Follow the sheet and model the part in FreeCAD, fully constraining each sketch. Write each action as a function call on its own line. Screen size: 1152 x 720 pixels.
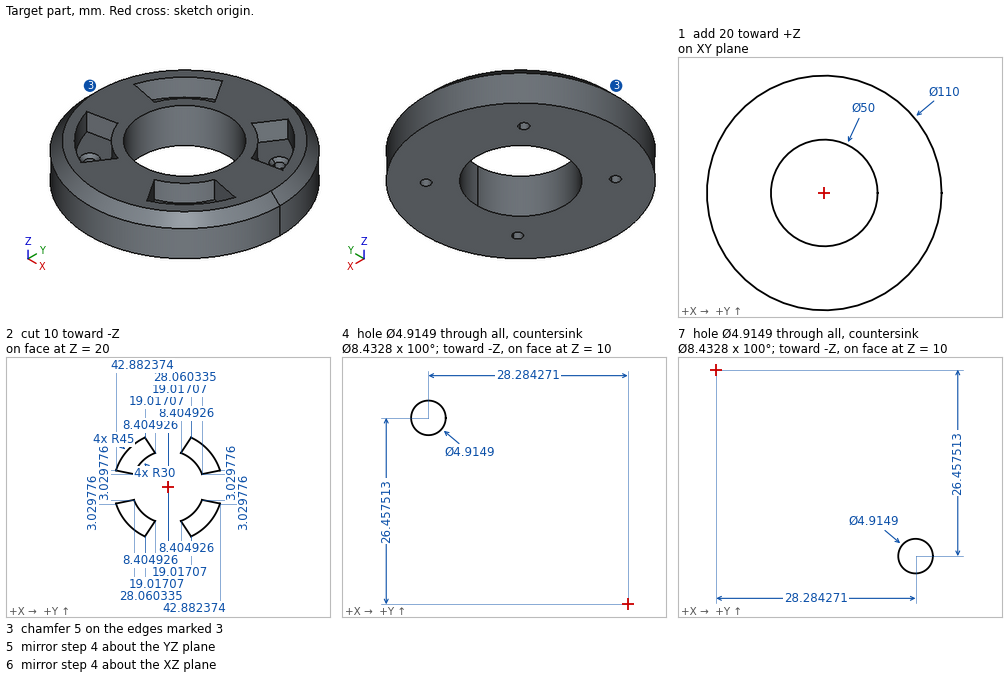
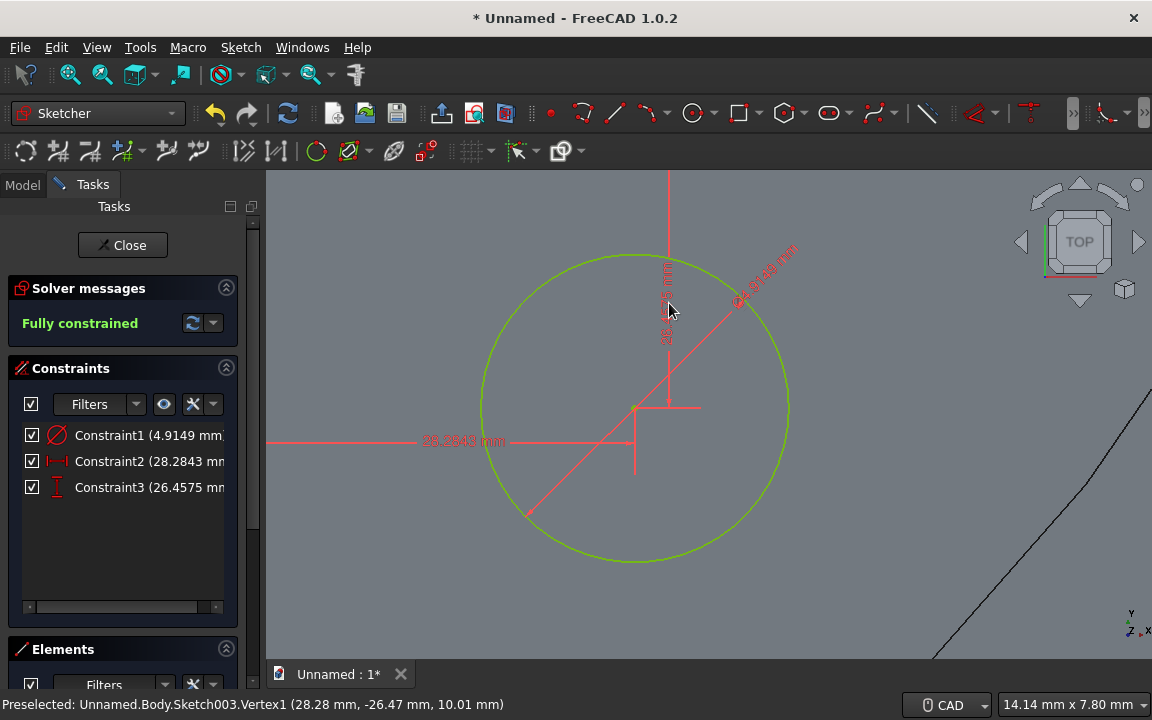
click(123, 245)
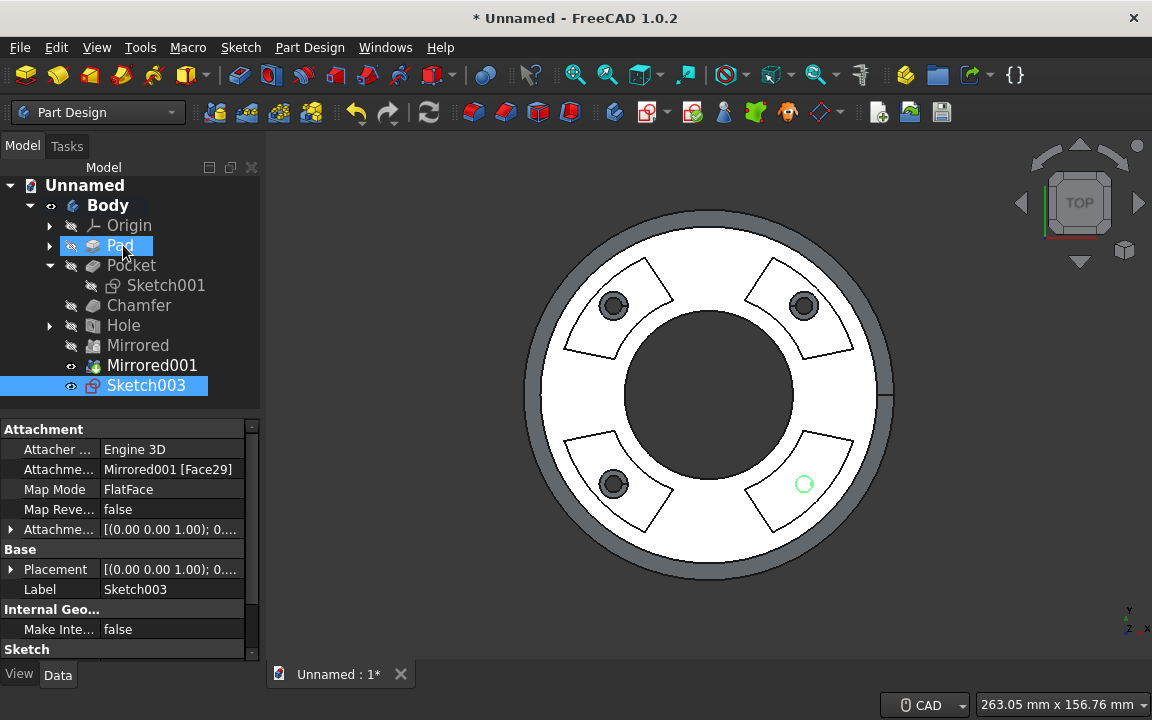
click(272, 76)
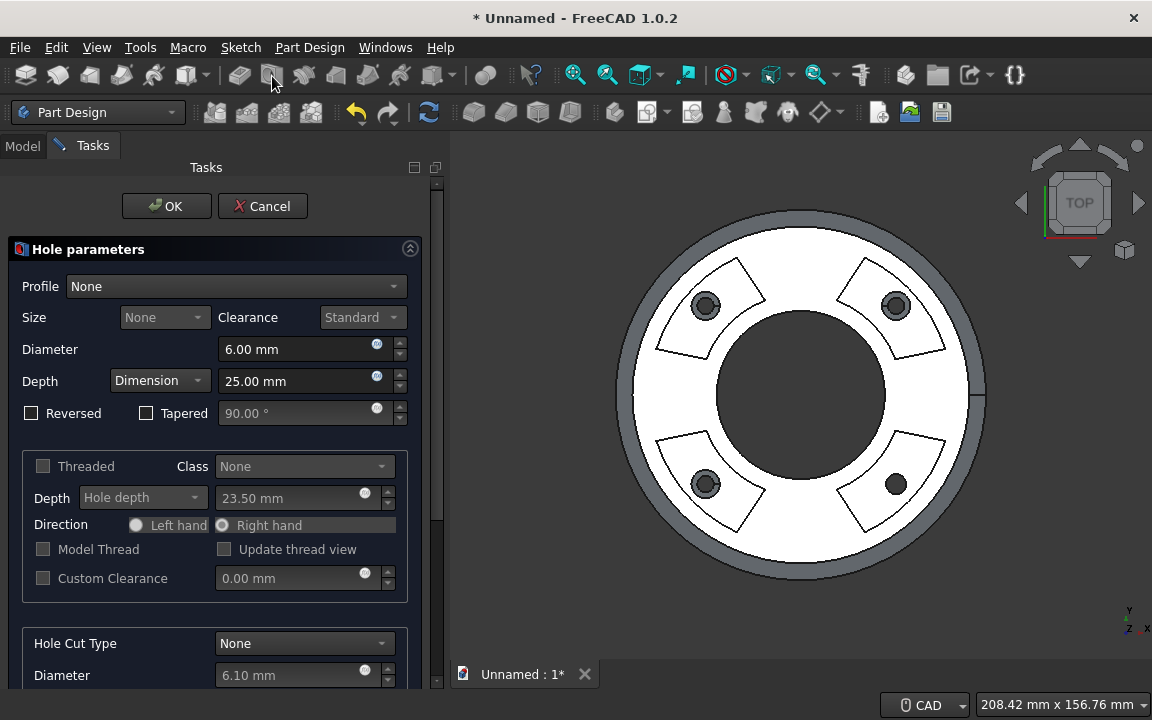
triple_click(305, 349)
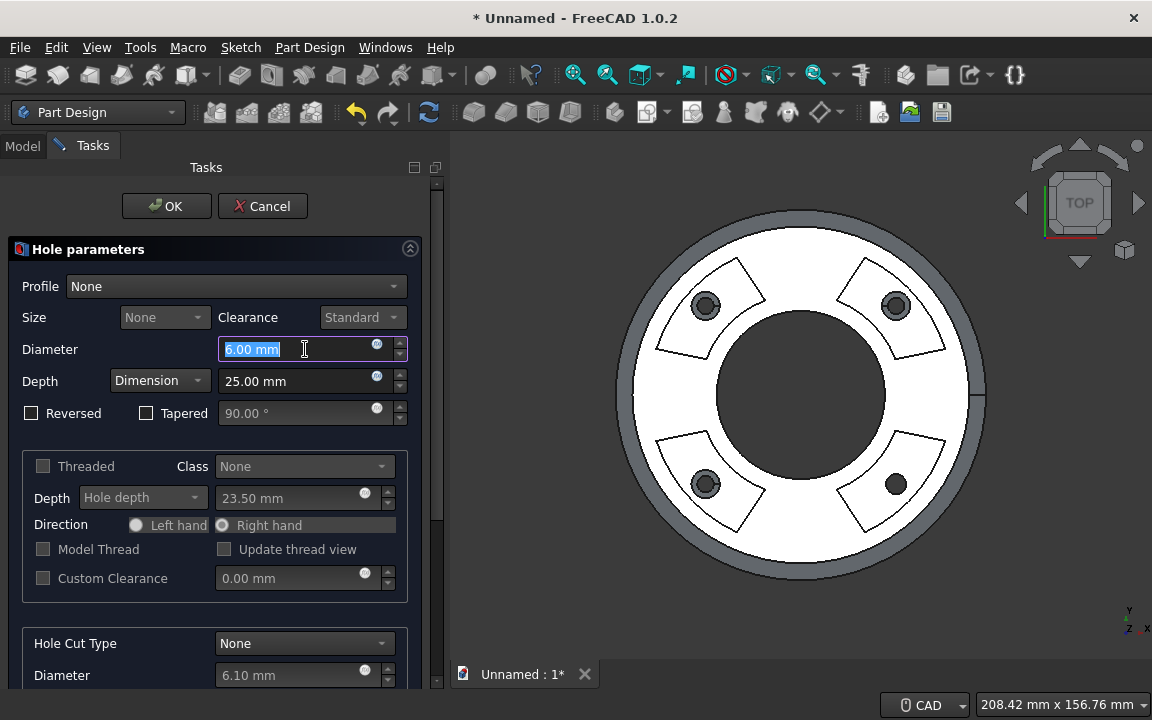
text(4.9149)
key(Tab)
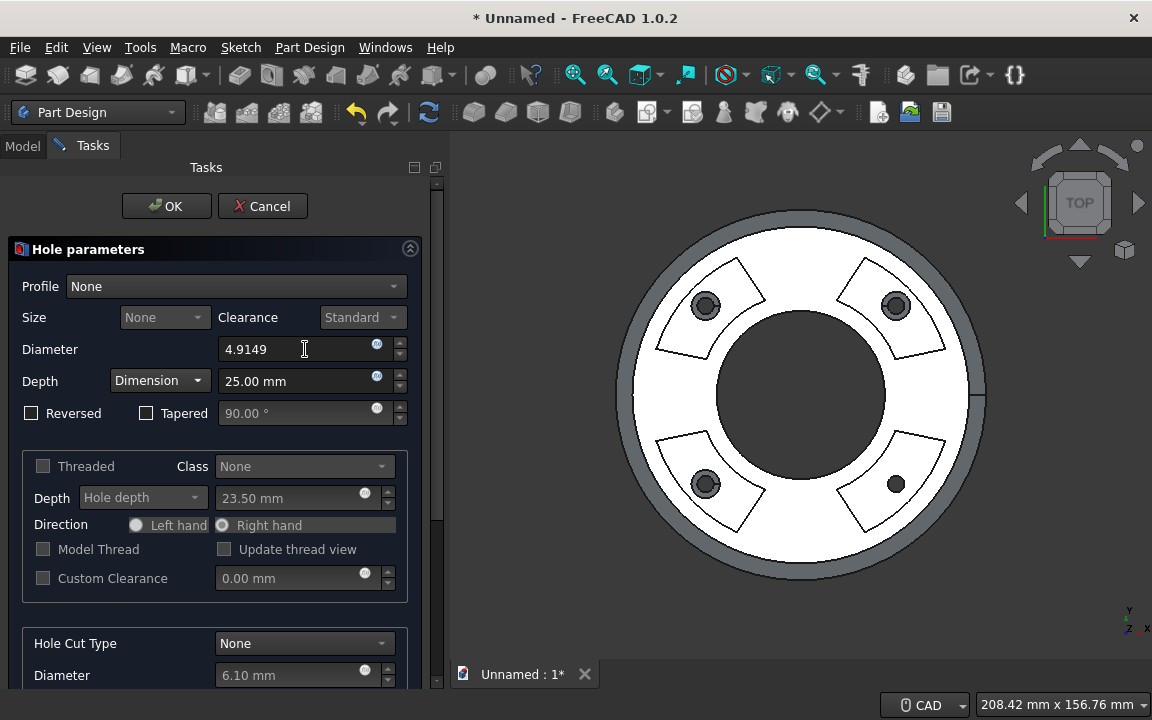
click(161, 380)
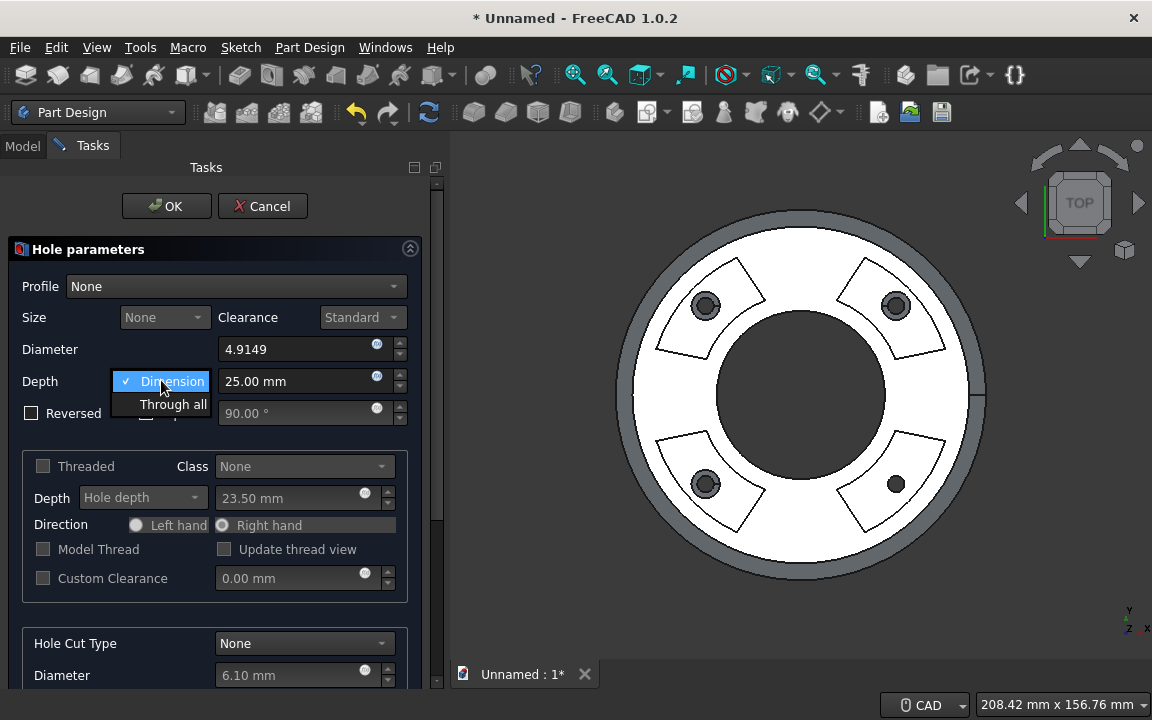
click(160, 404)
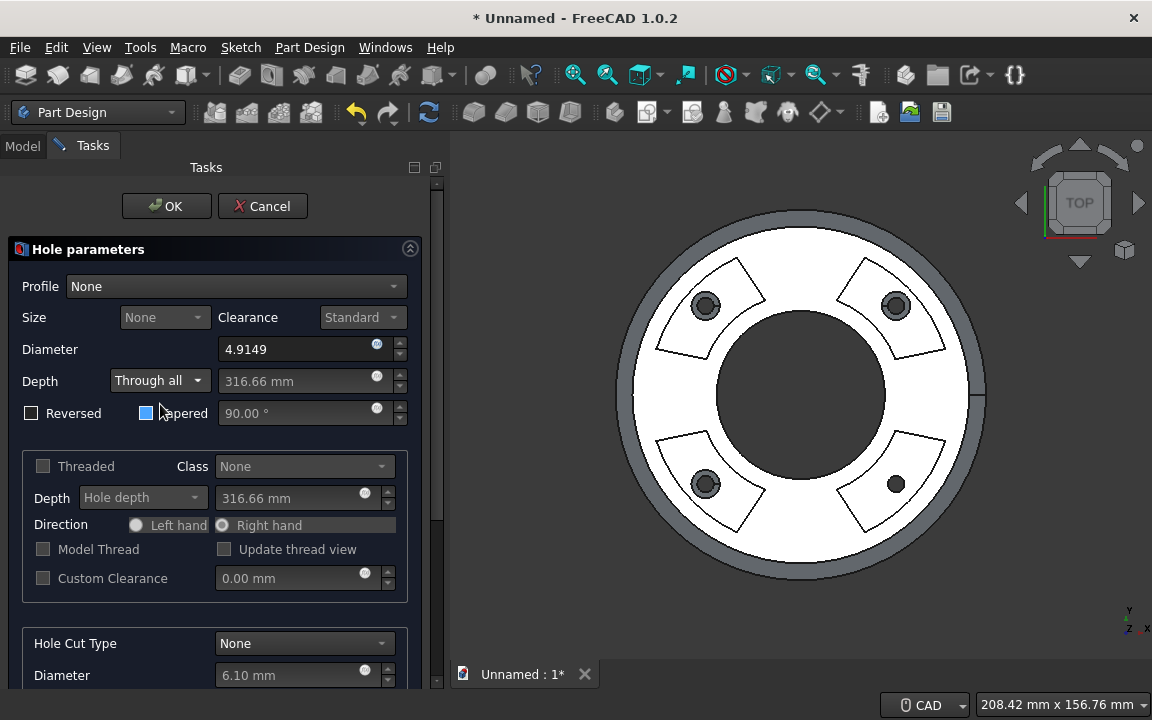
click(306, 644)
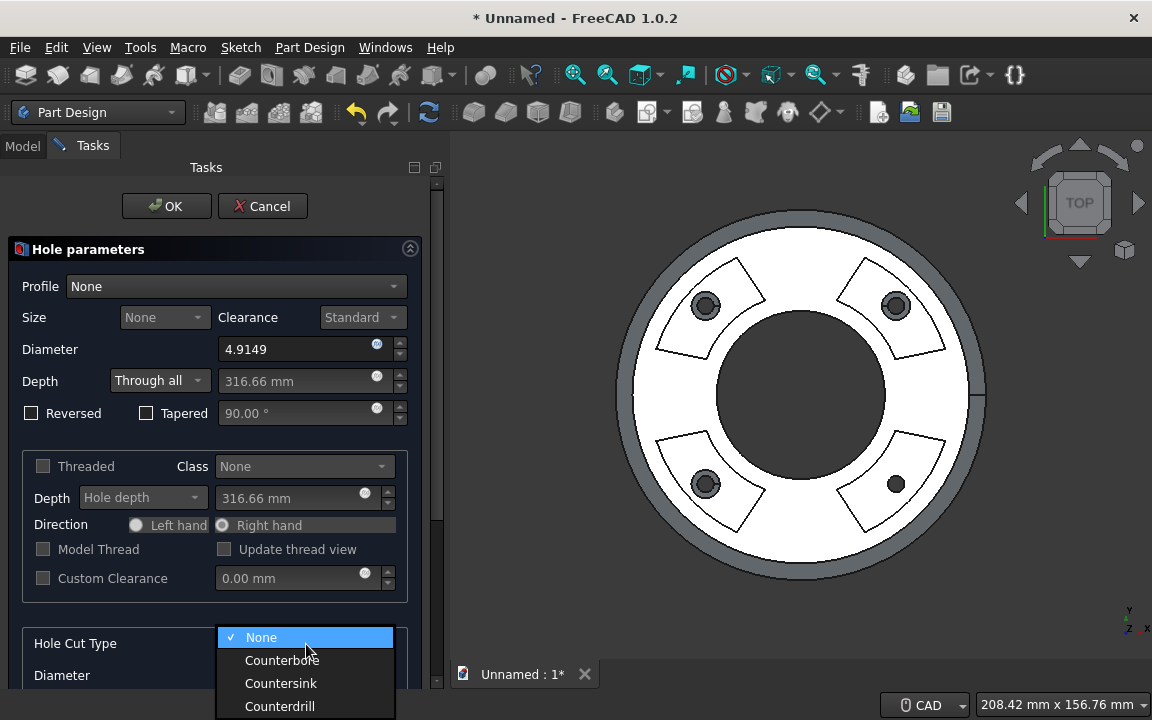
click(304, 684)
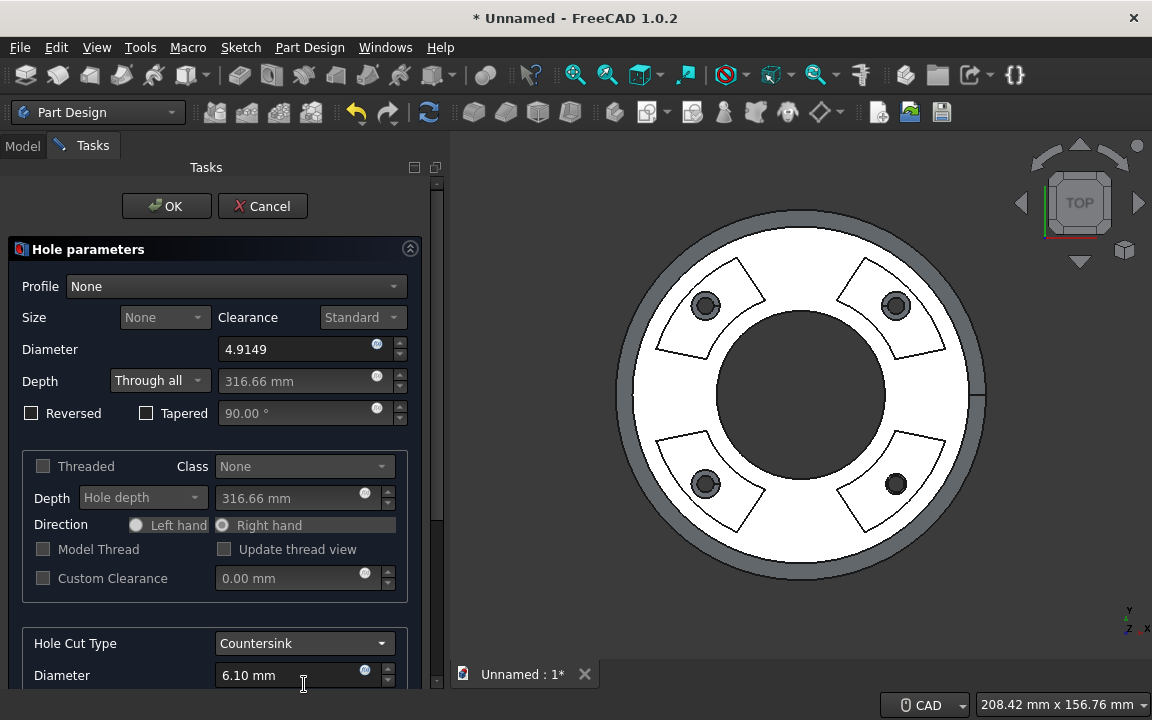
scroll(437, 432, down, 3)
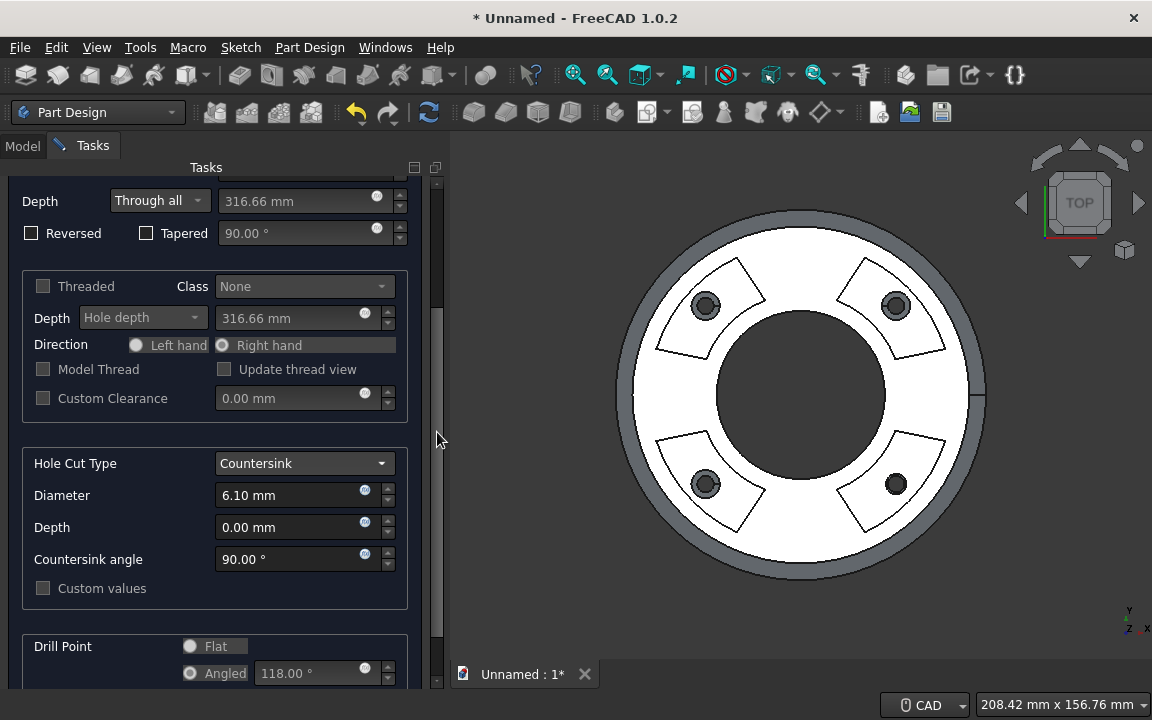
triple_click(298, 559)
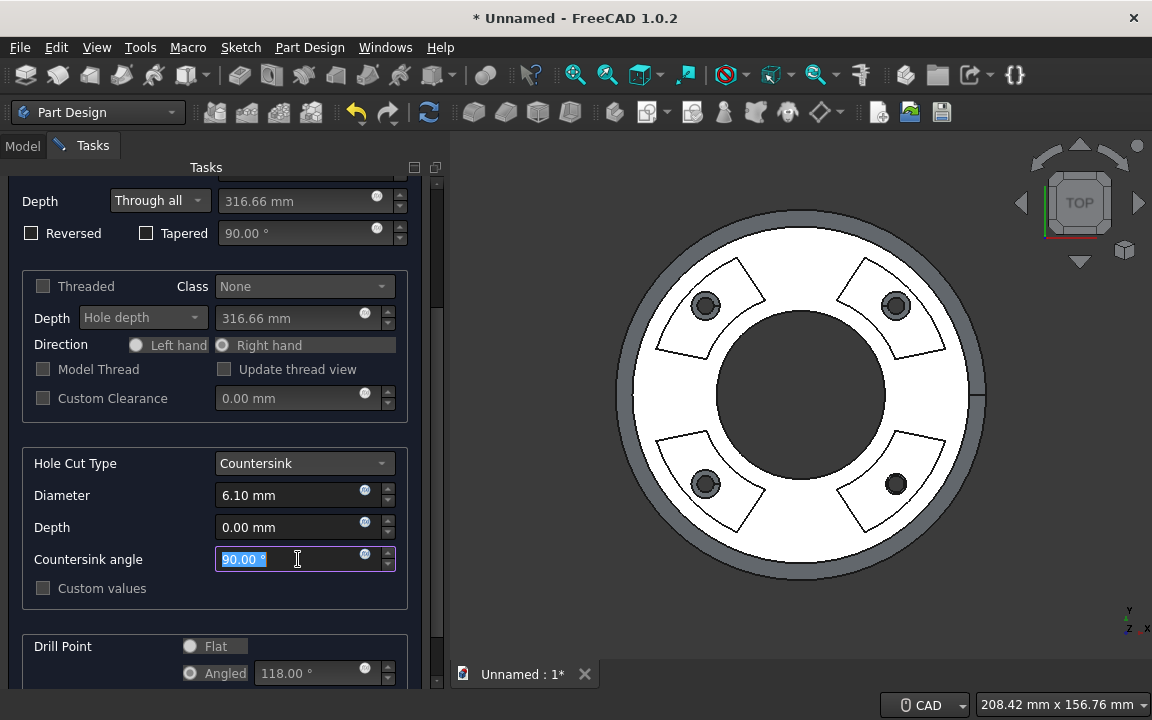
text(100)
key(Tab)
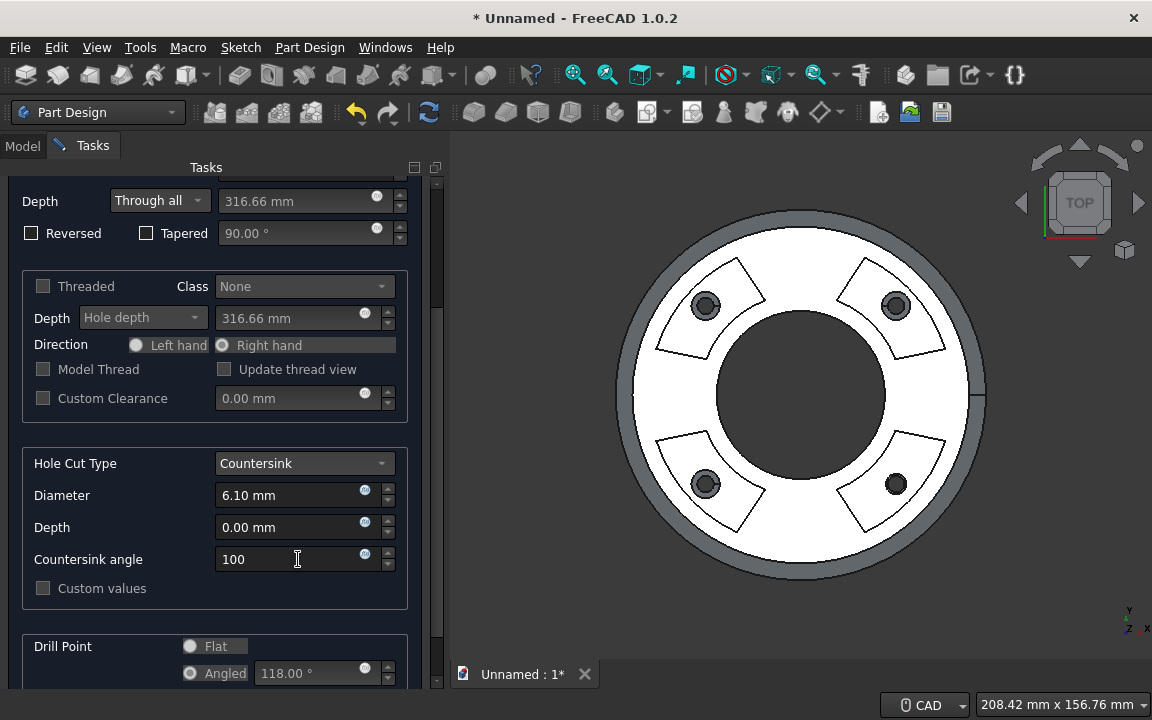
triple_click(298, 495)